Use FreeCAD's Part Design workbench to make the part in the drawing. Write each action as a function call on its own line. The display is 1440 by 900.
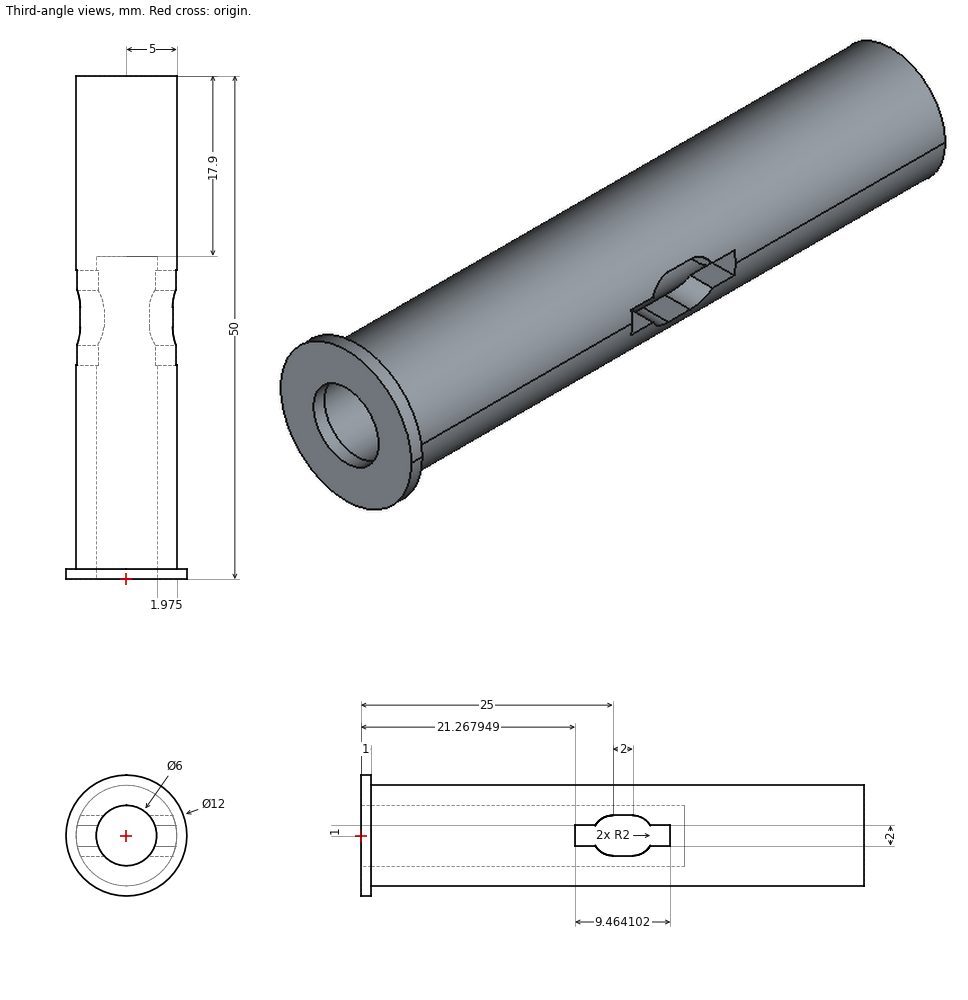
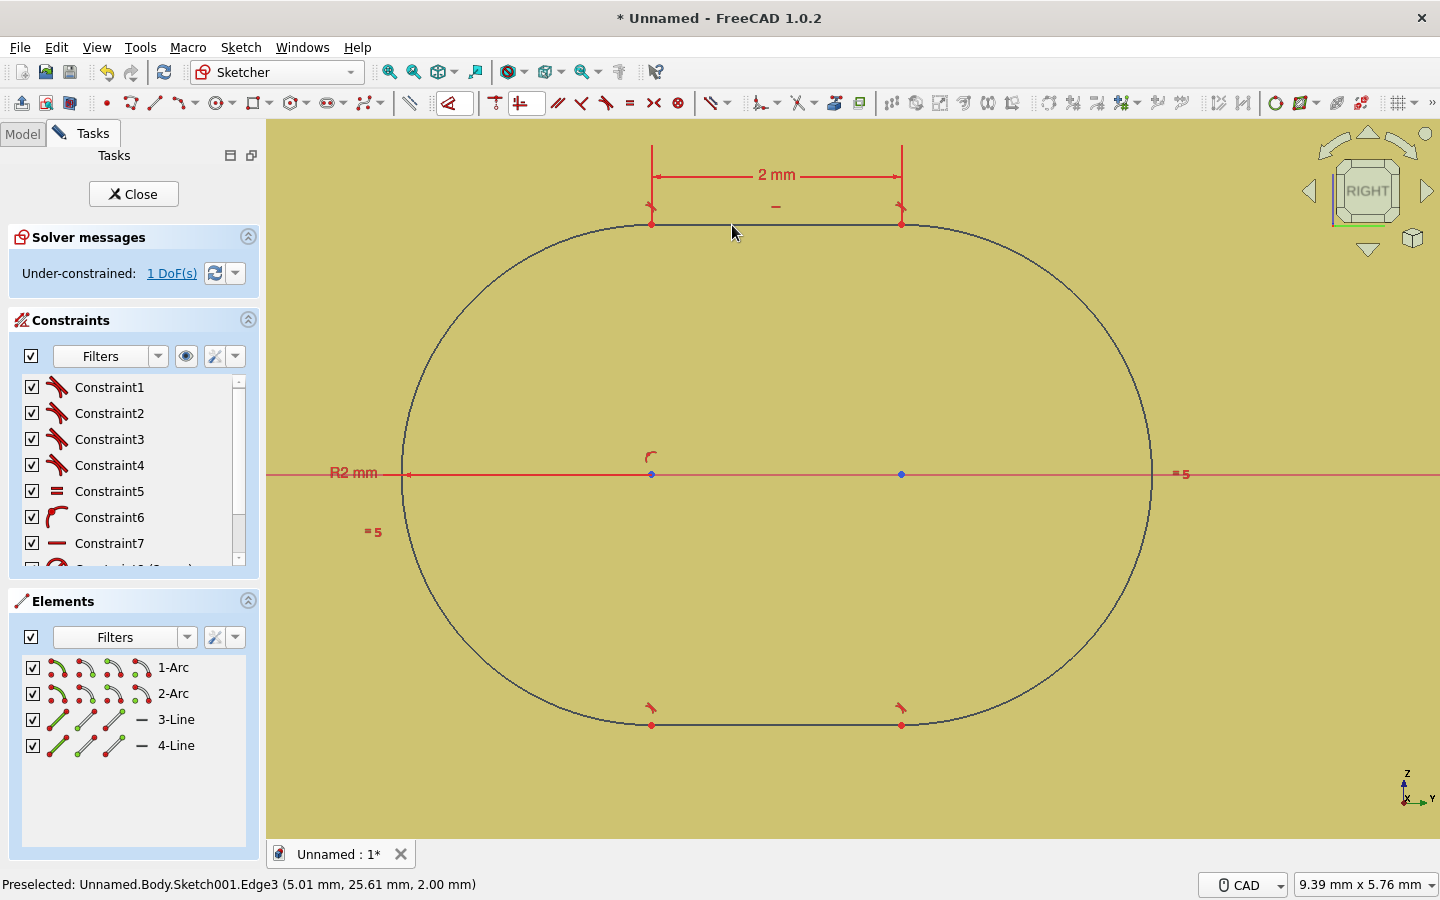
click(652, 225)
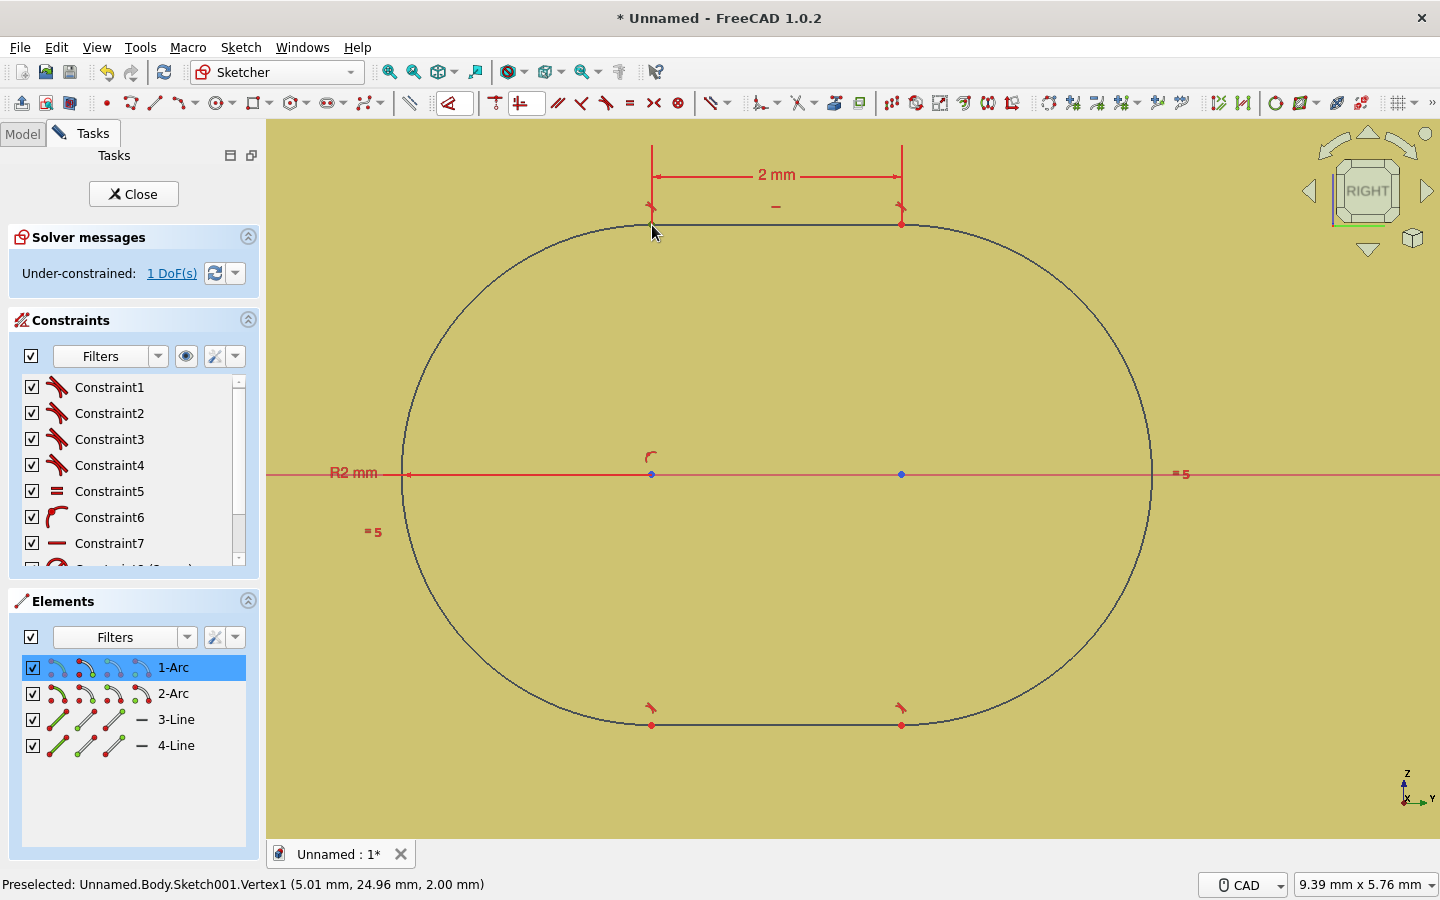
key(l)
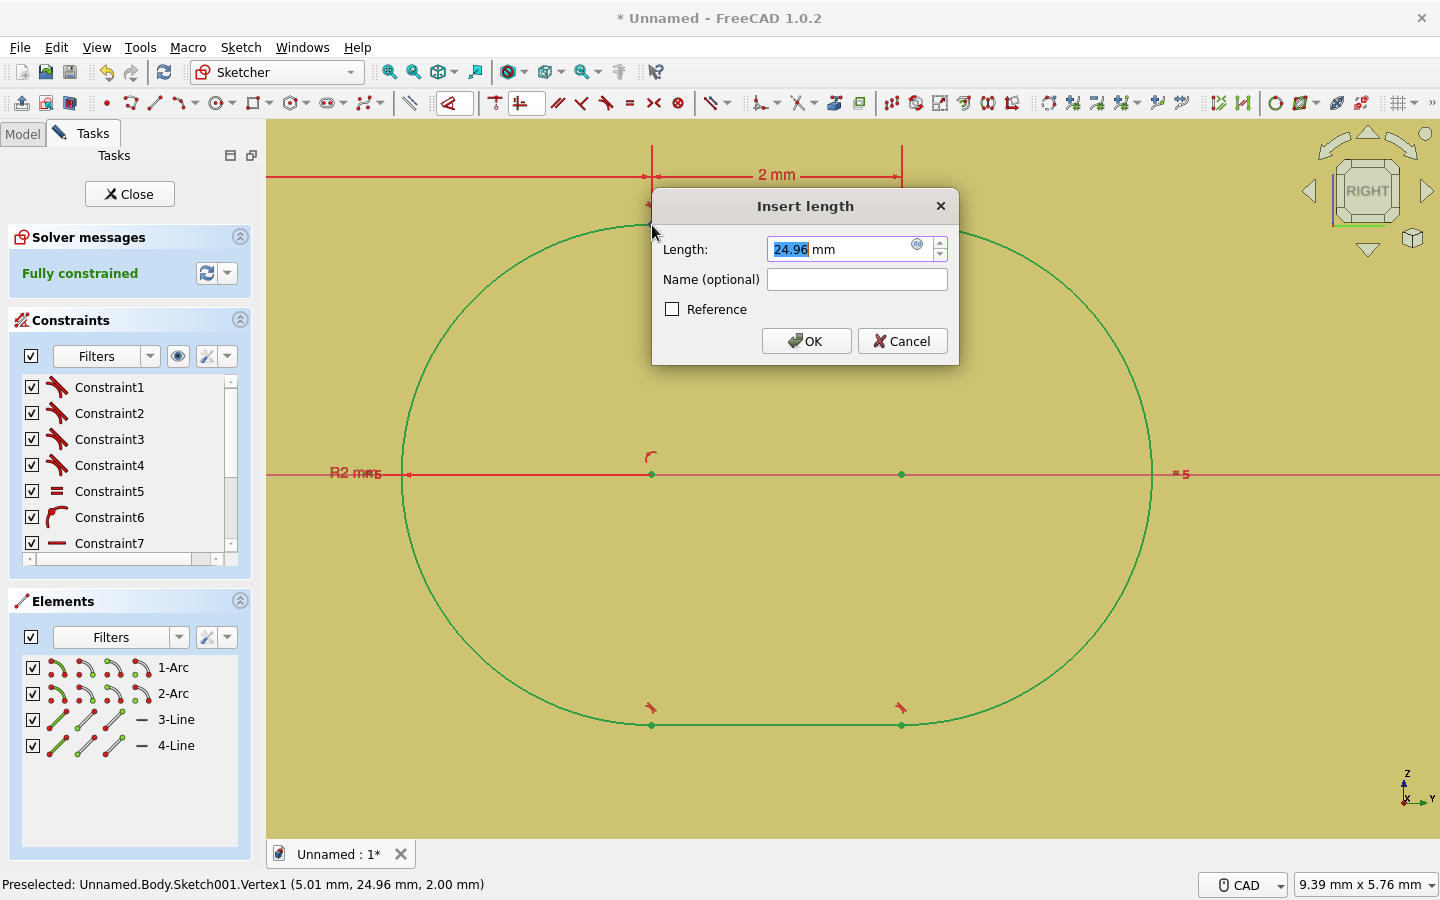
text(25)
key(Return)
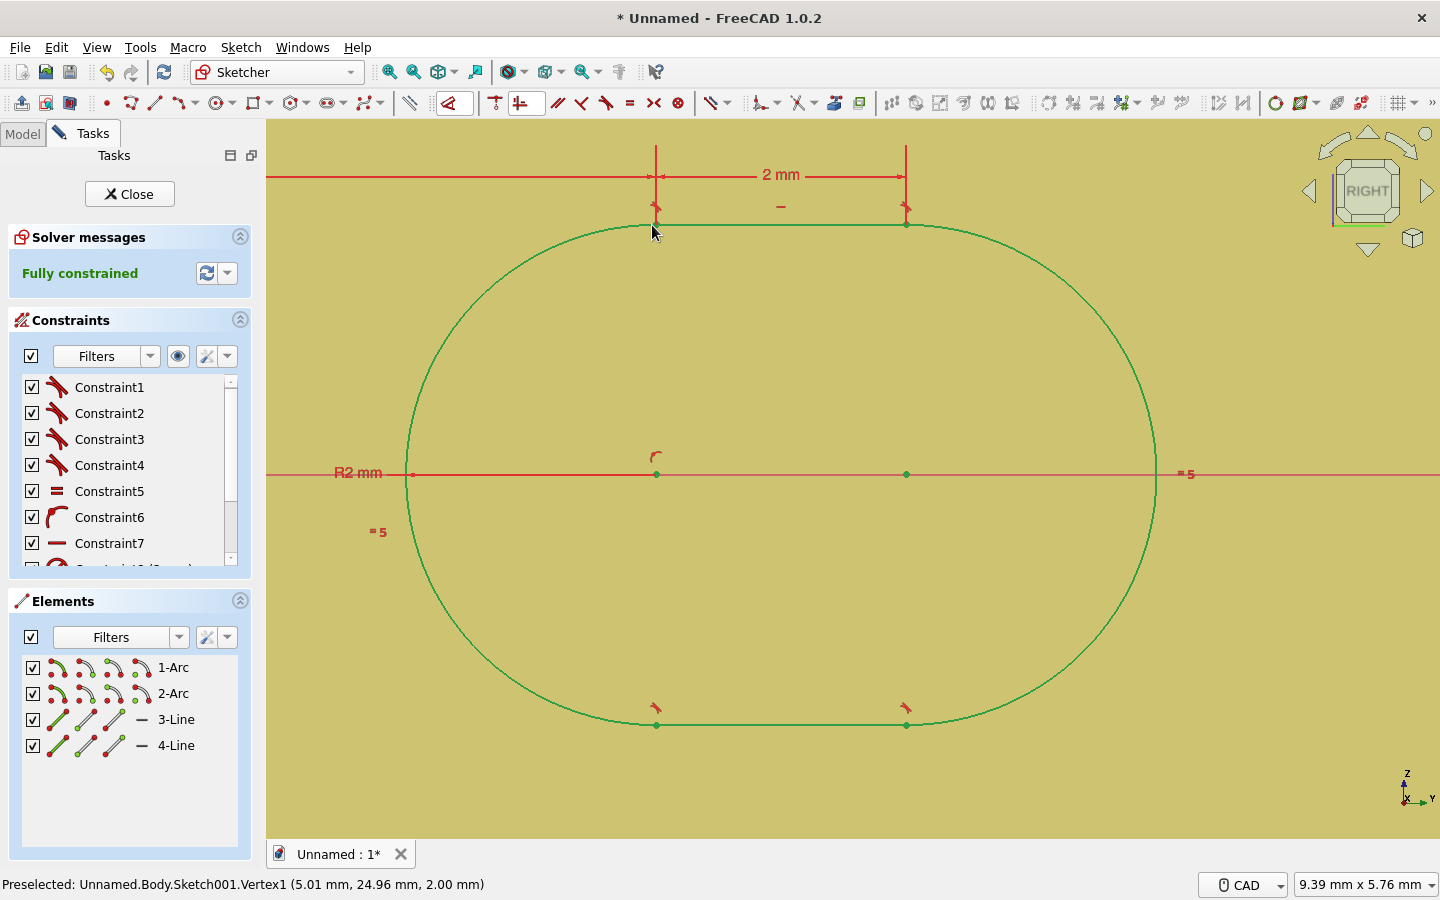
click(130, 194)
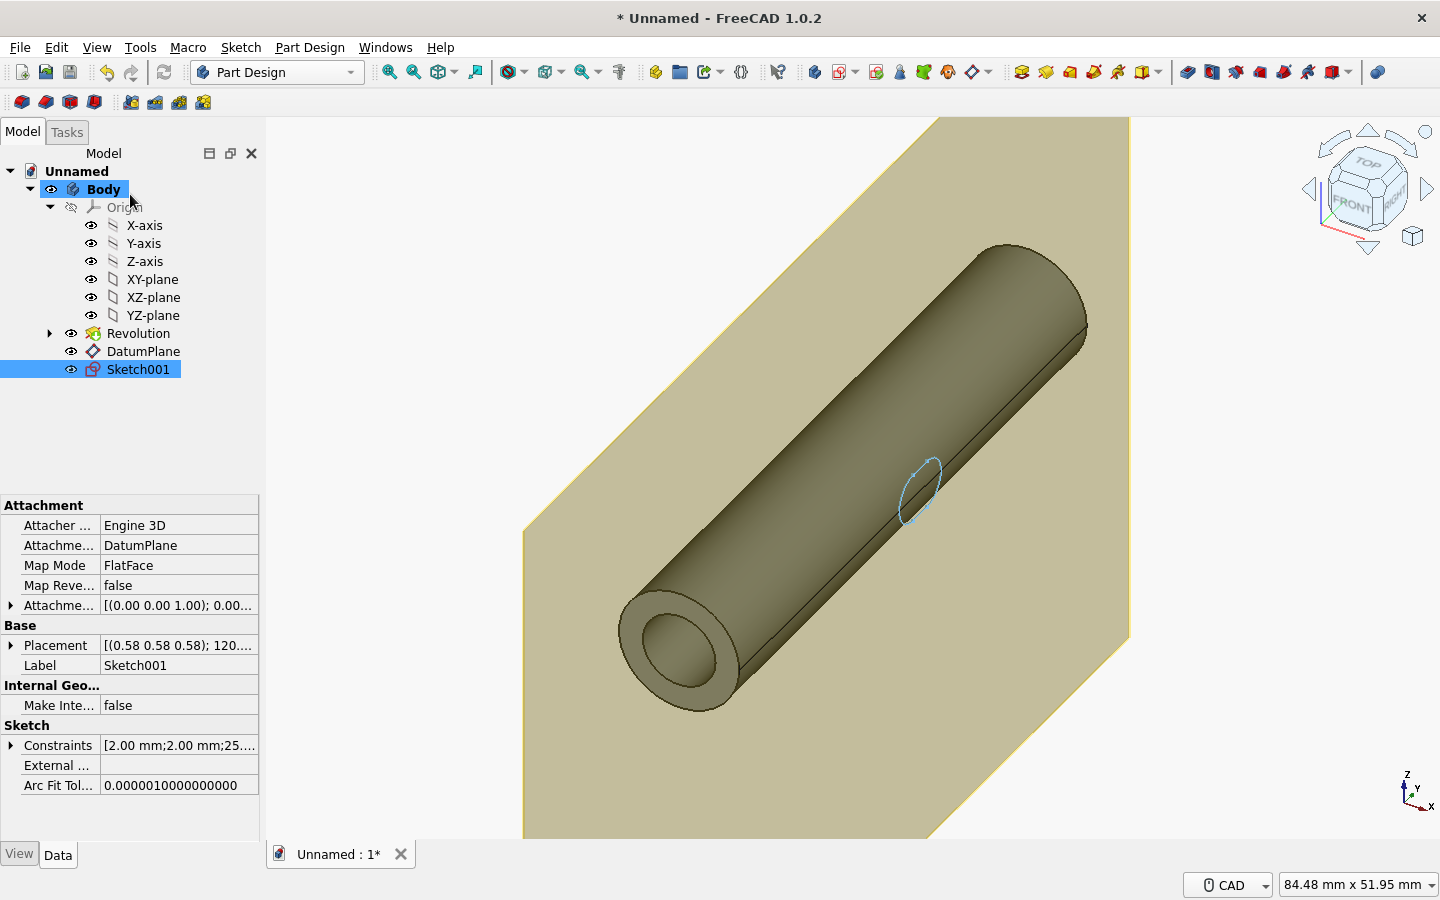
click(1188, 72)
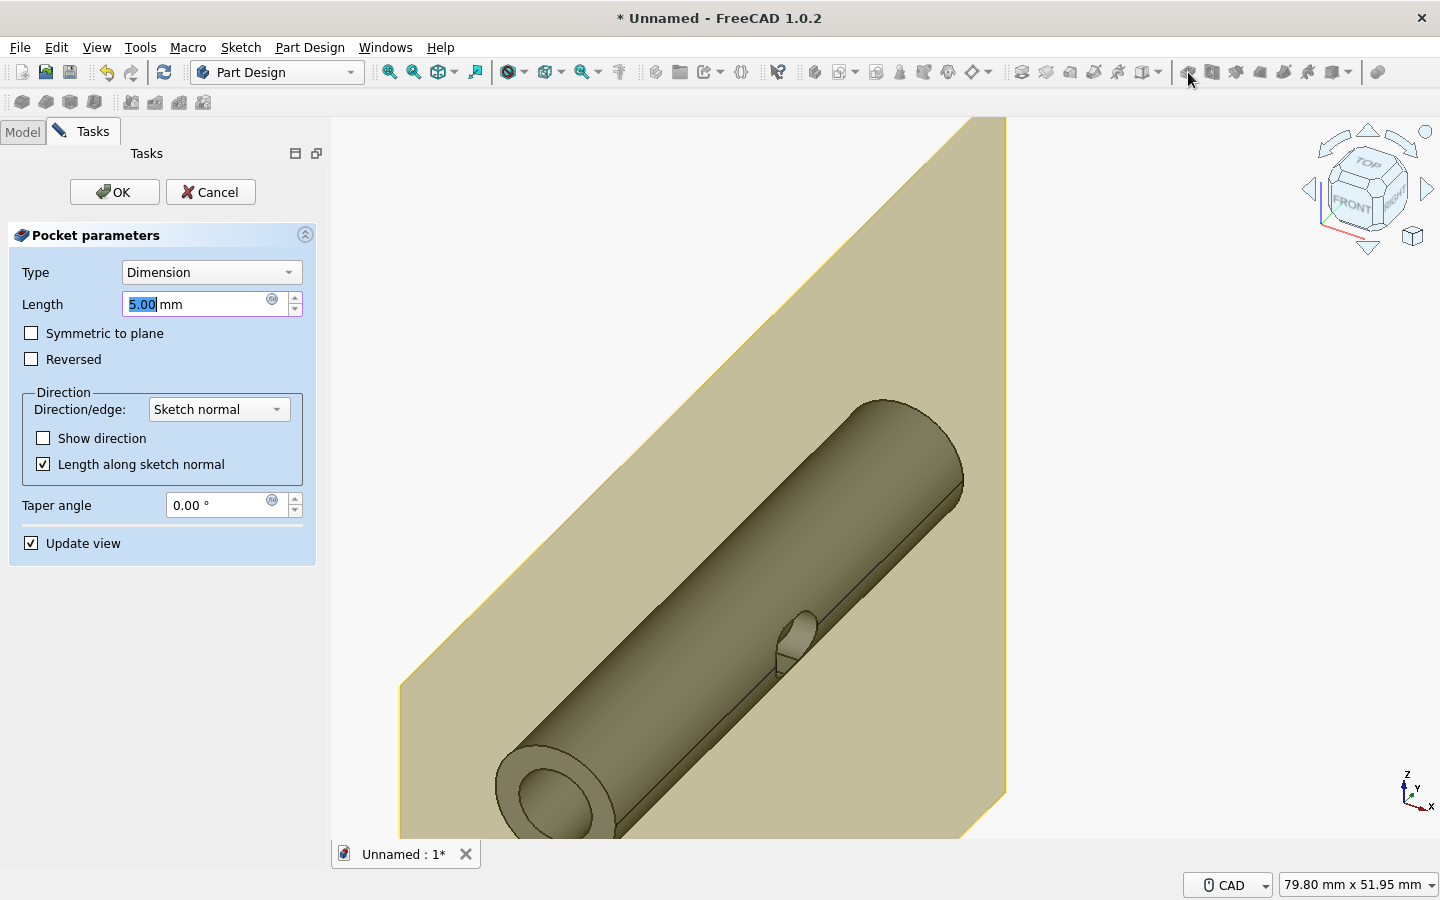
click(212, 272)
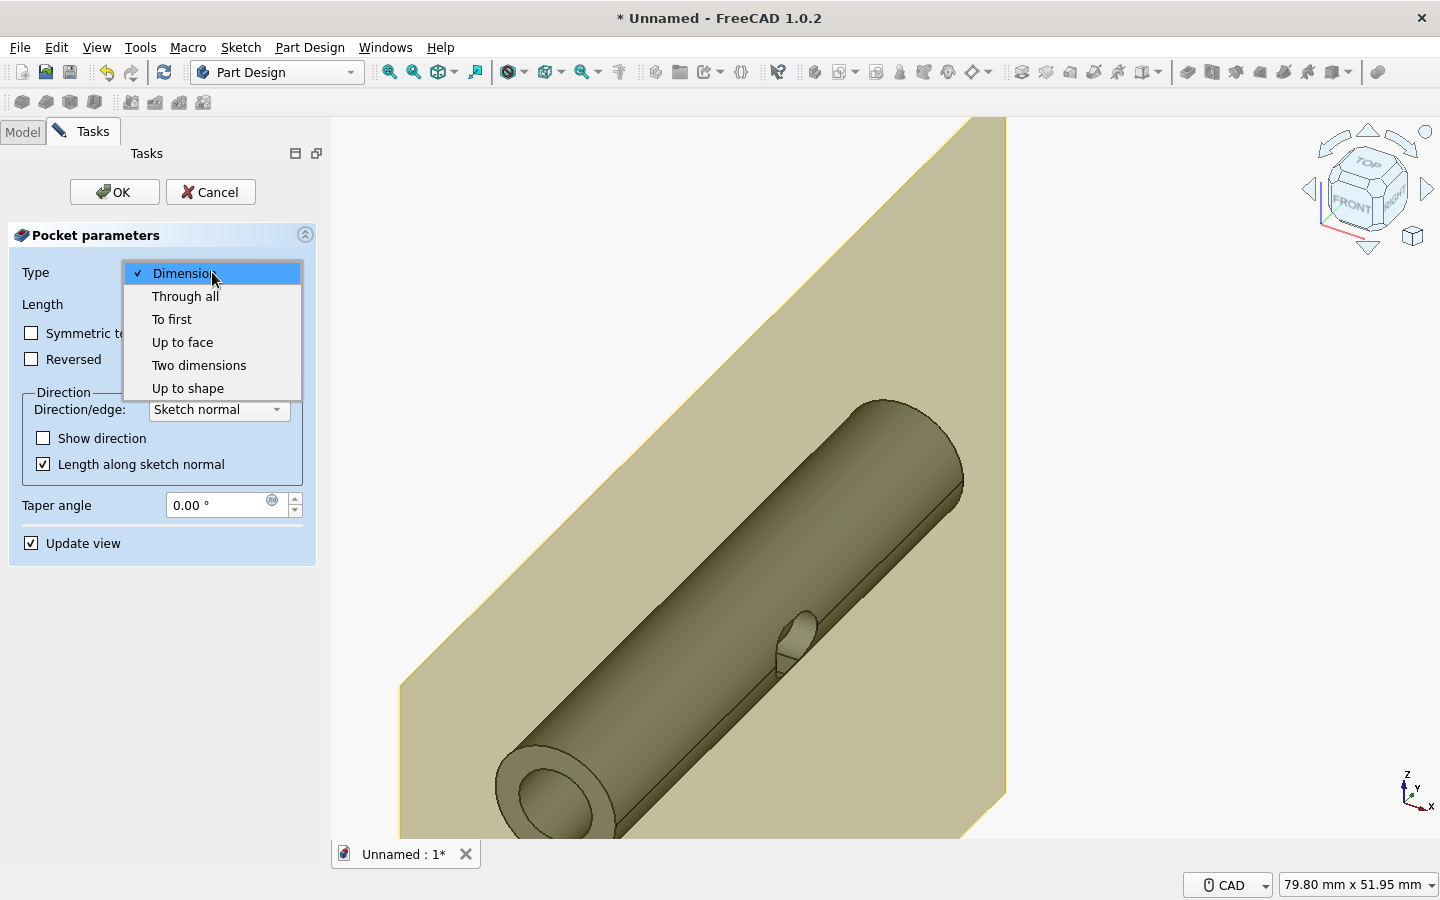
click(212, 296)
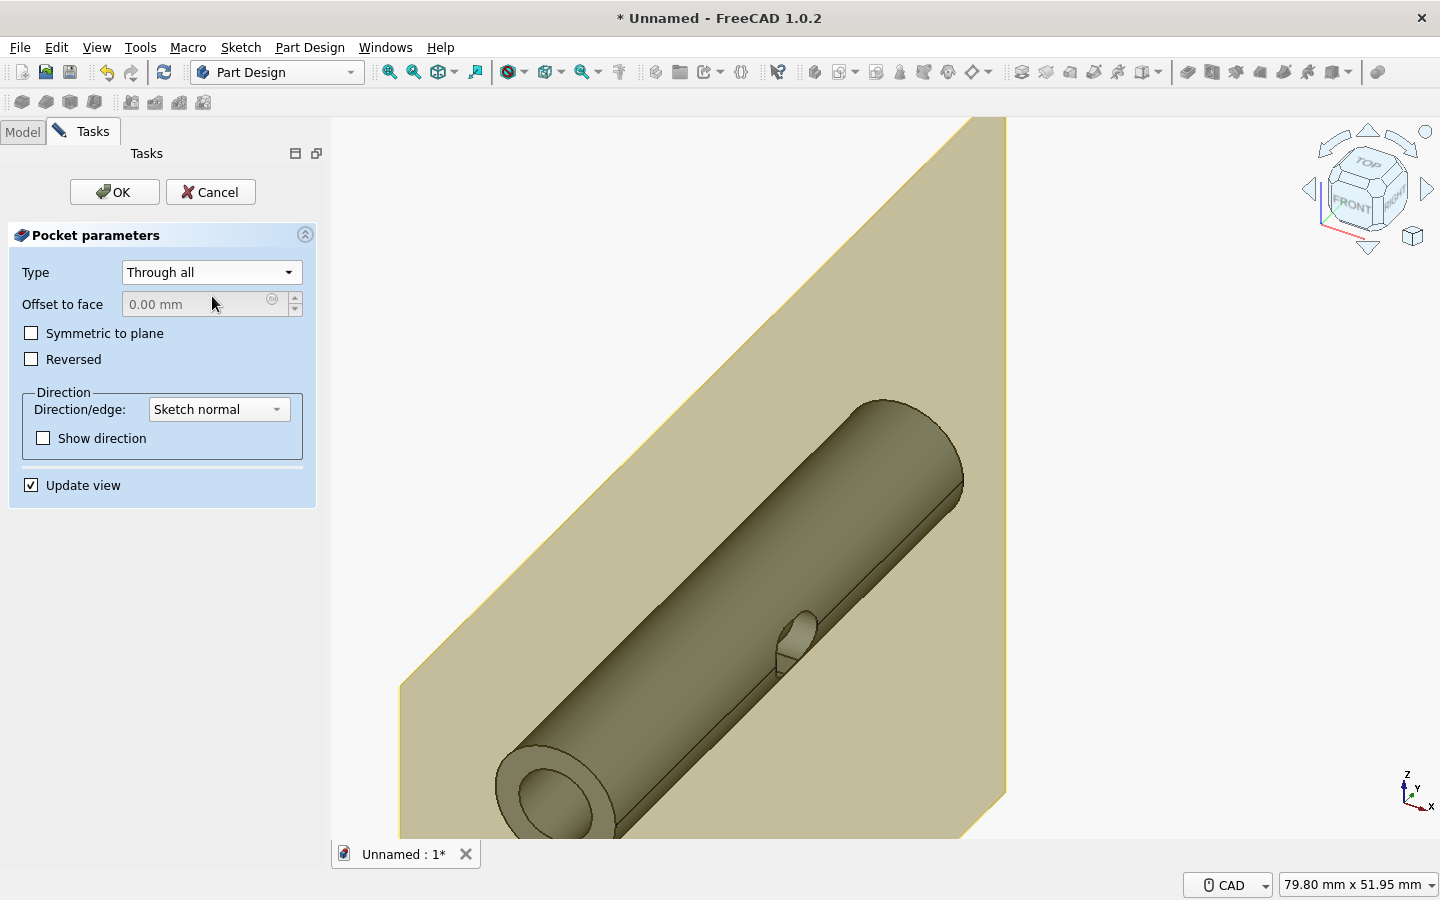
click(115, 192)